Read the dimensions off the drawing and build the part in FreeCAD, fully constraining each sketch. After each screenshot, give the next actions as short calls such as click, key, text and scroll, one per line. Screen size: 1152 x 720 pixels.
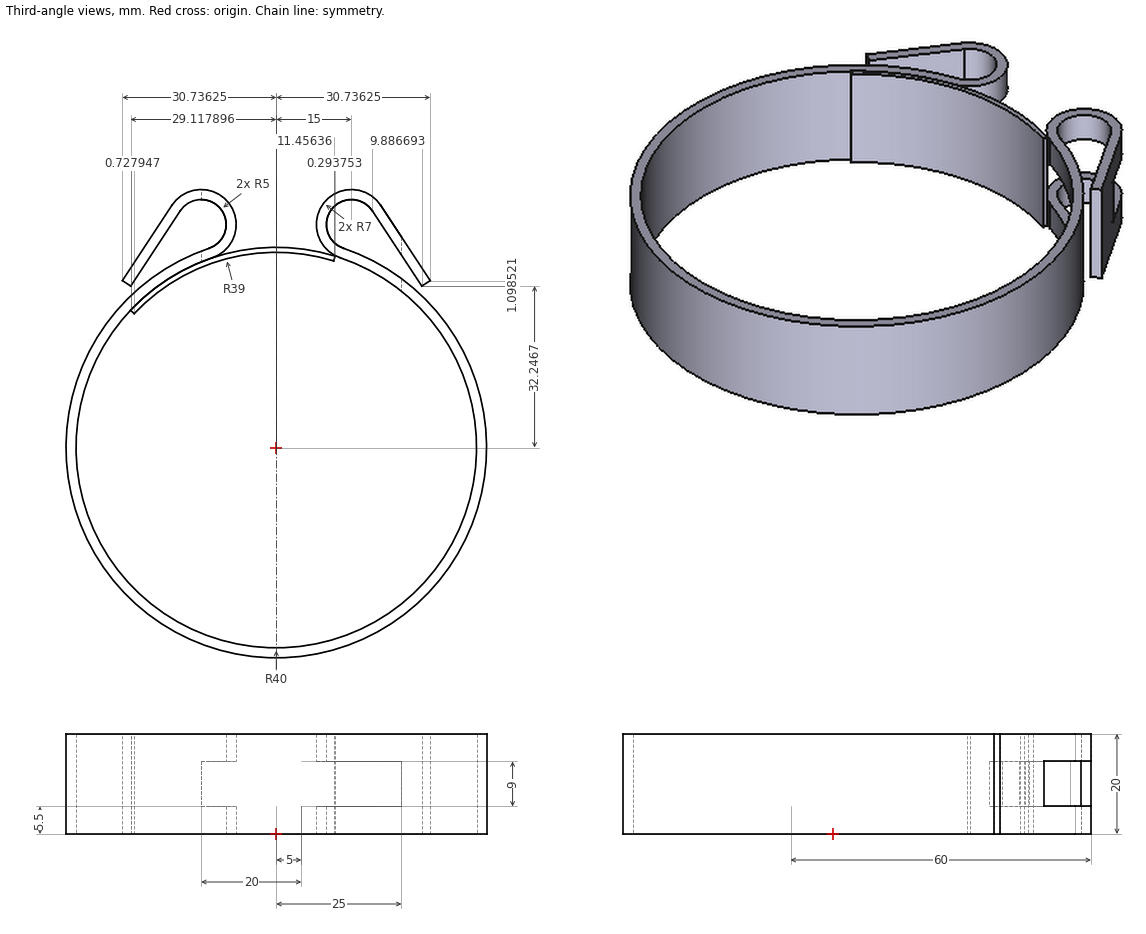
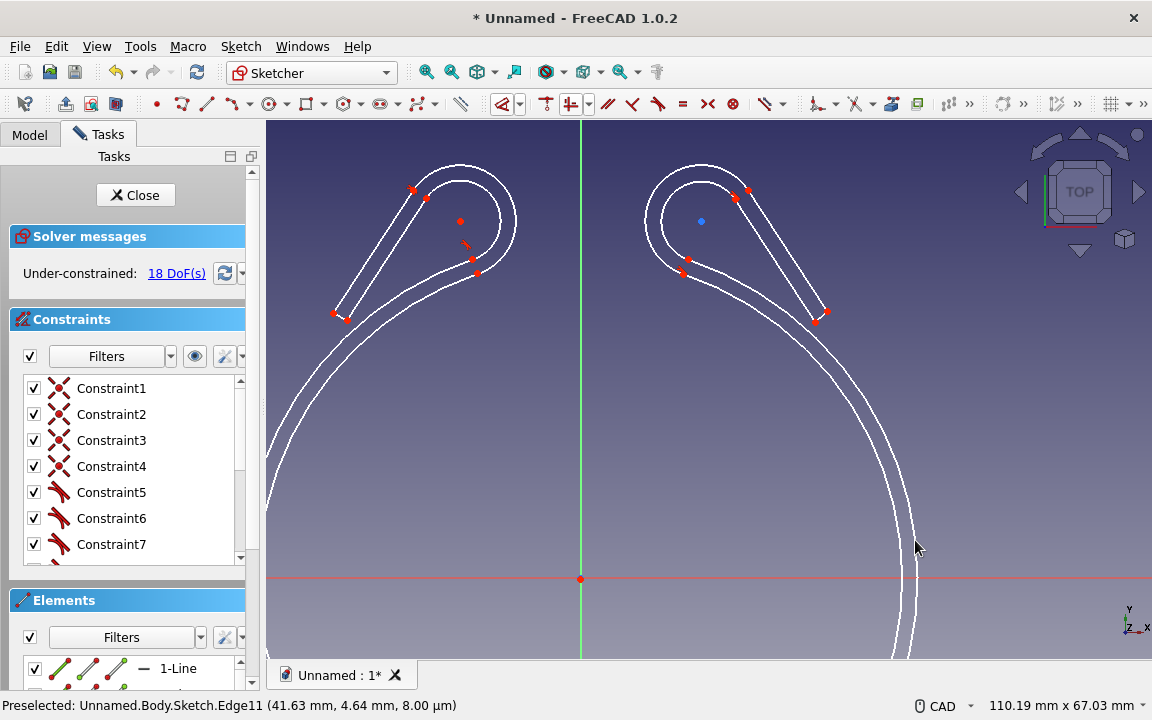
click(693, 166)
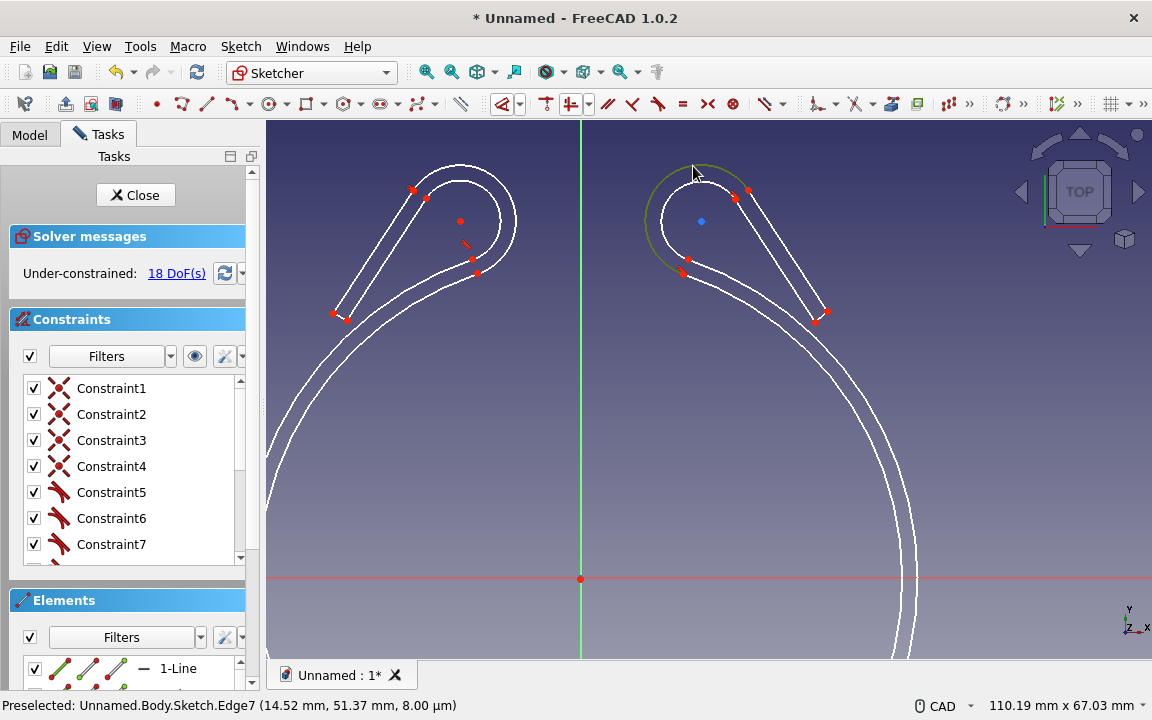
click(696, 182)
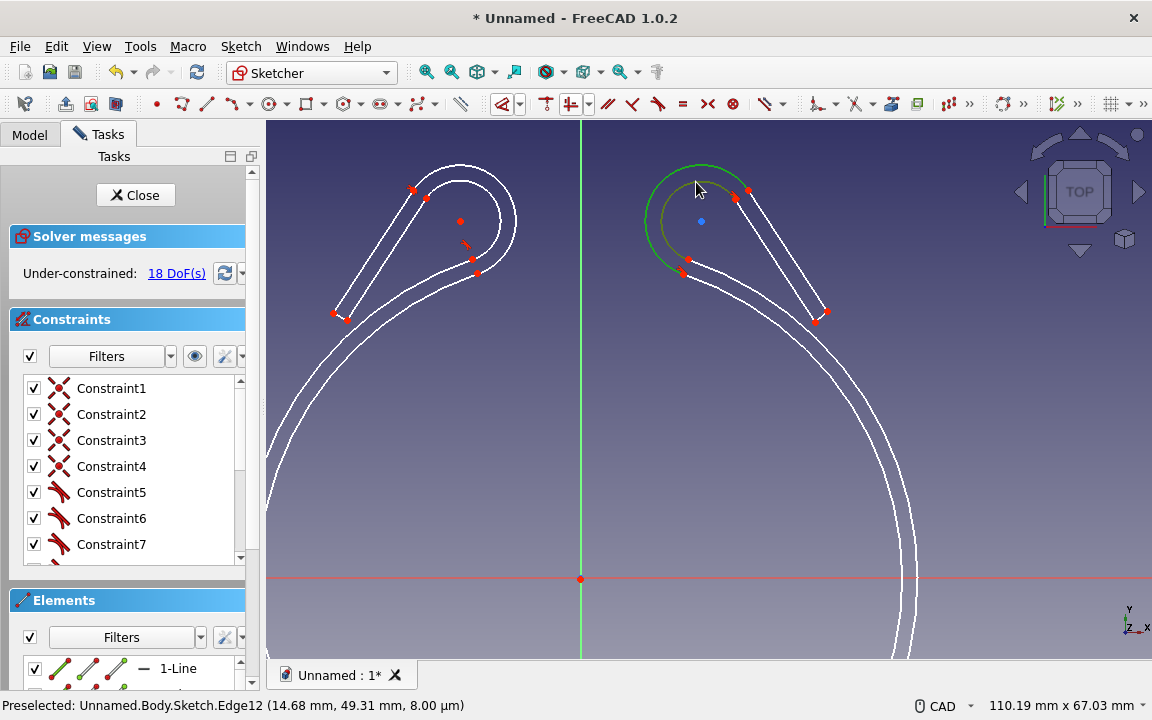
key(c)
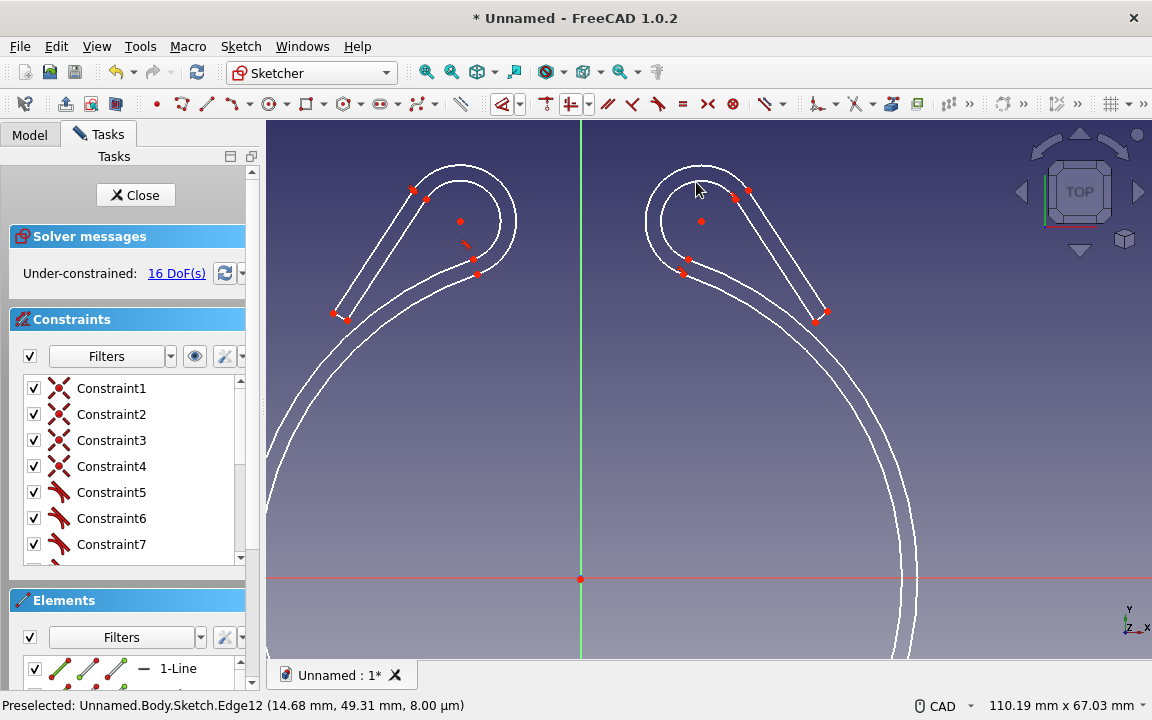
drag(570, 568, 591, 589)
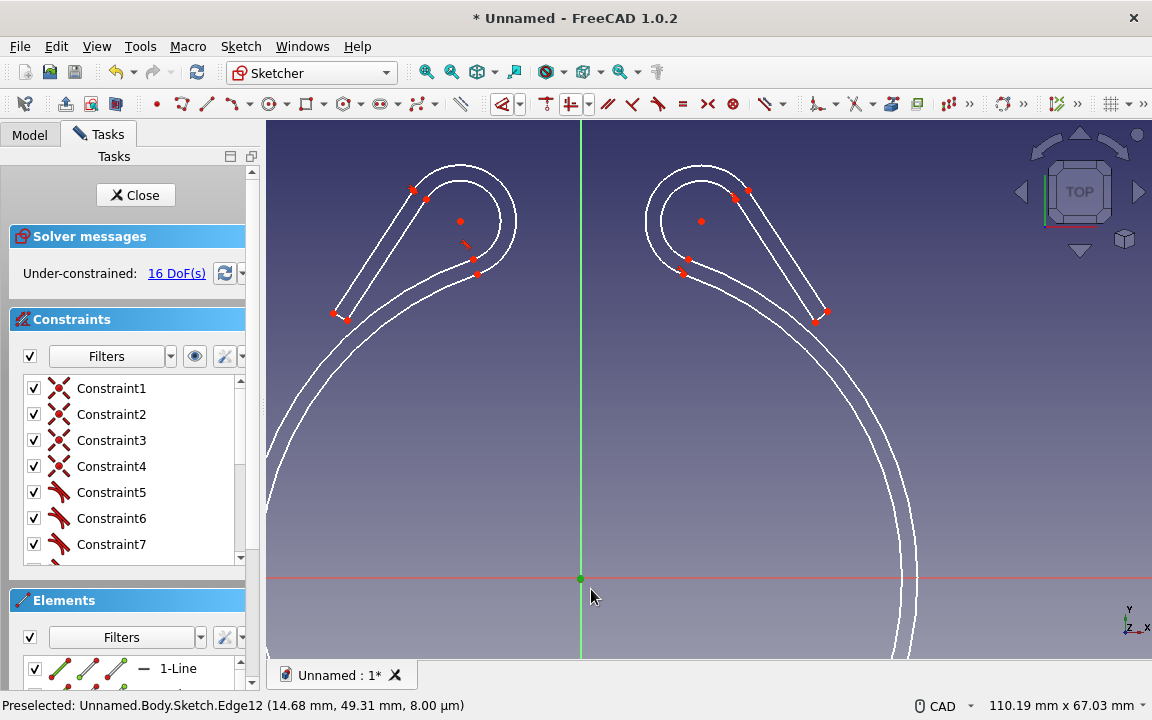
key(c)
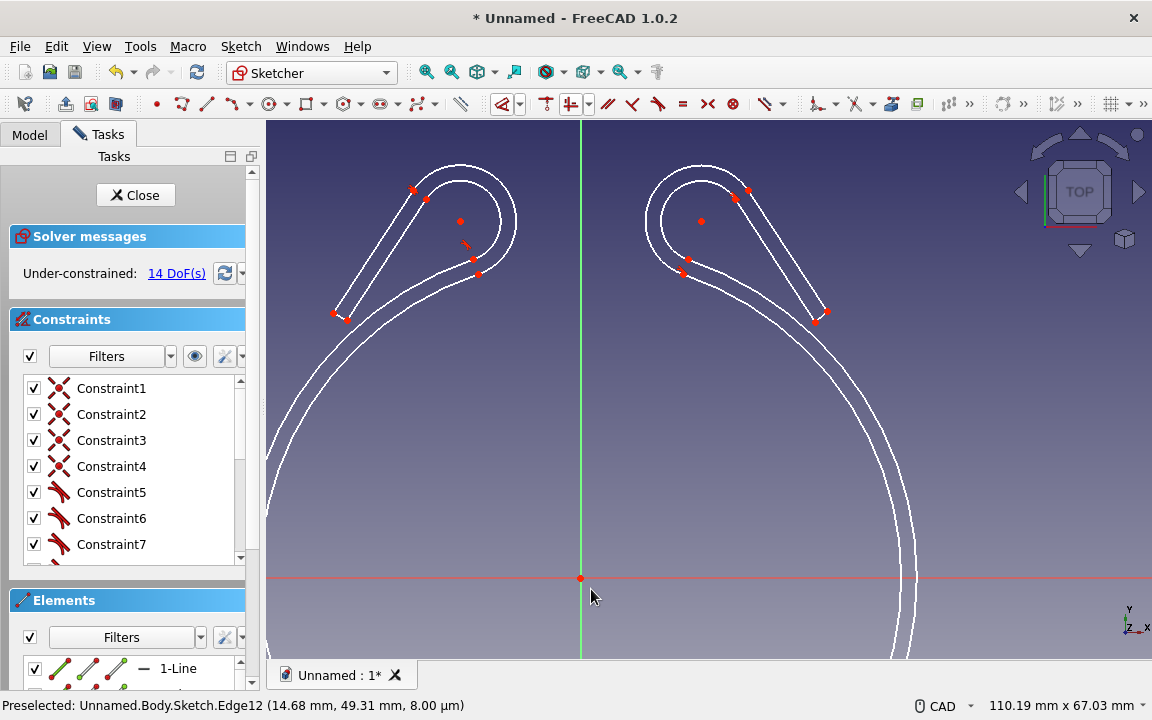
click(693, 166)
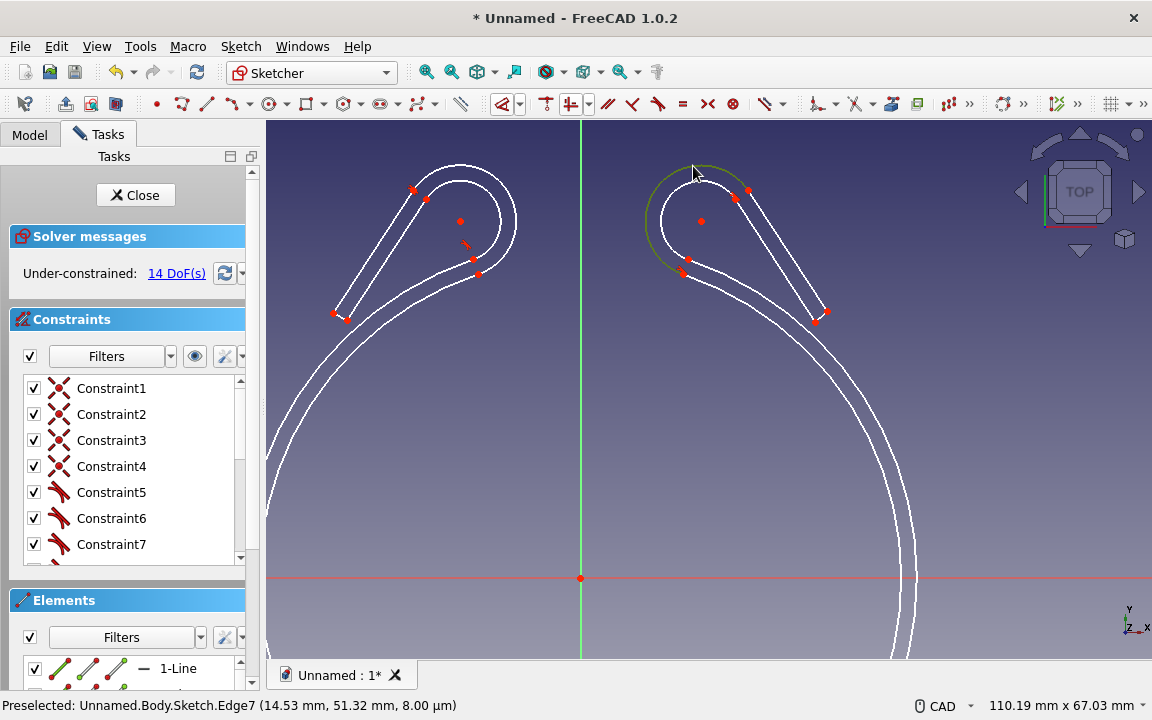
click(516, 227)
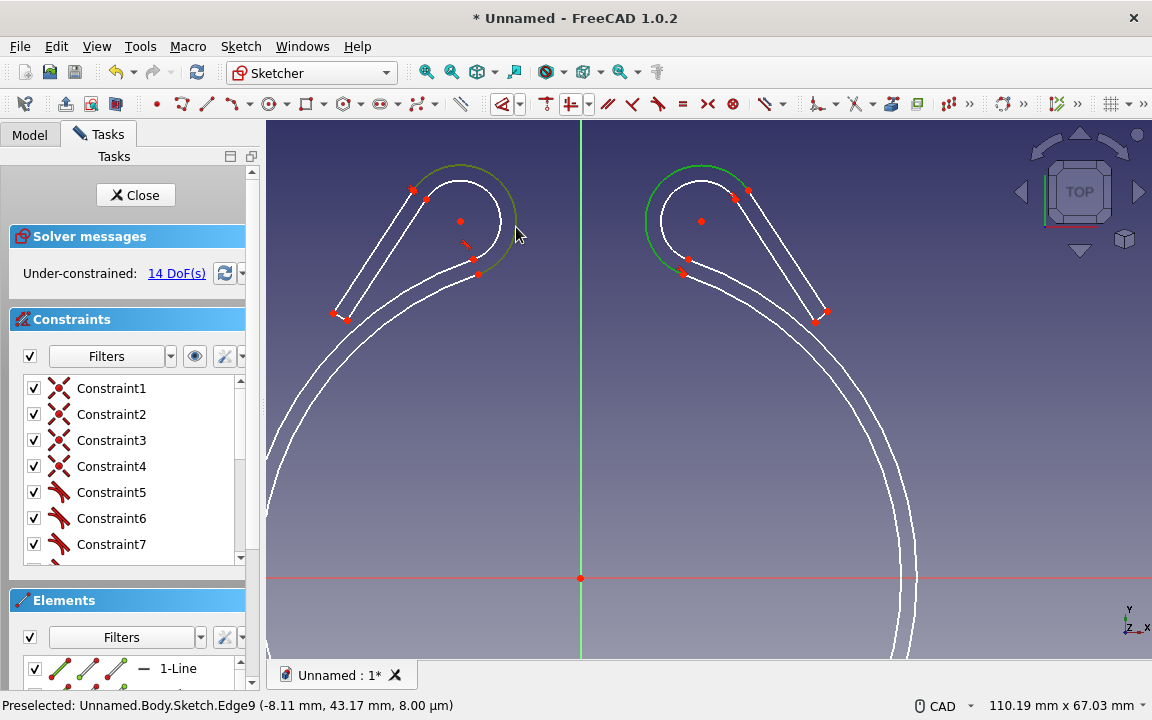
key(e)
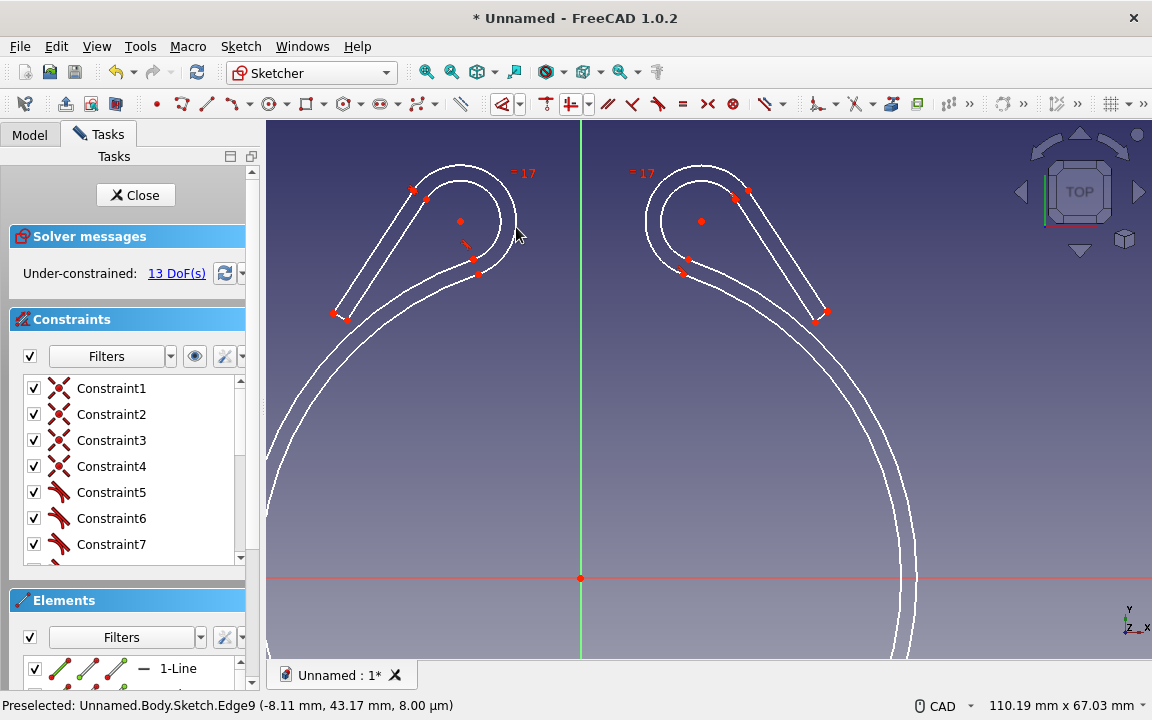
click(748, 191)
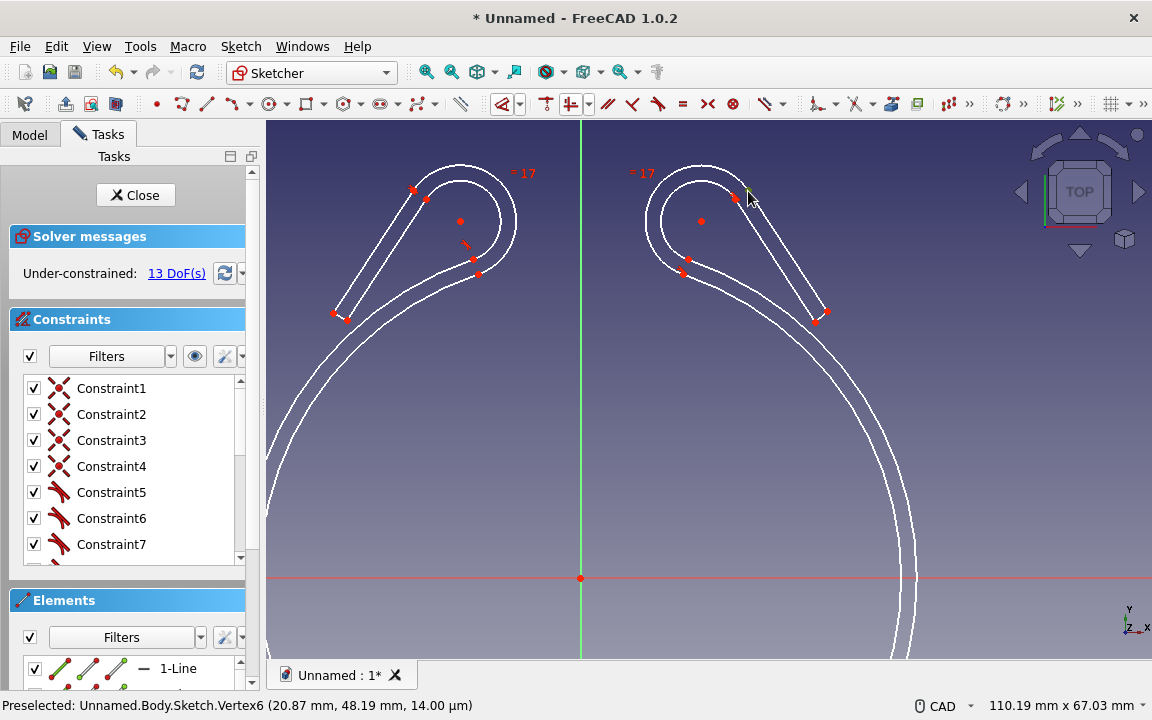
click(413, 191)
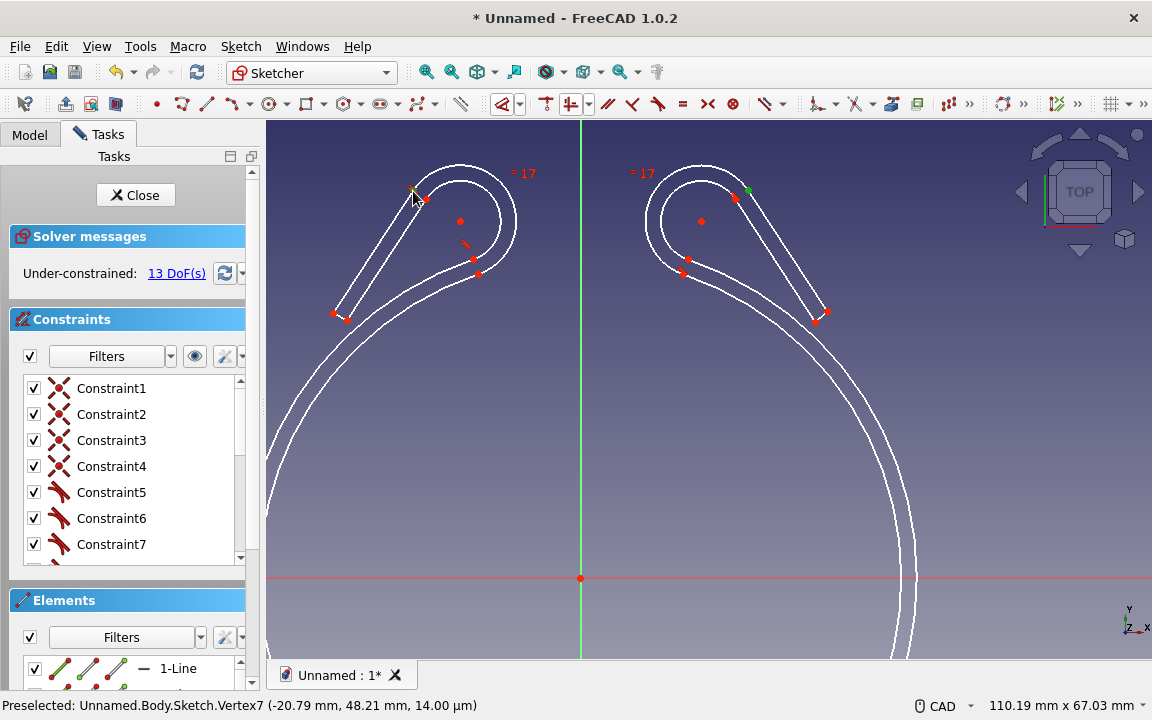
click(581, 528)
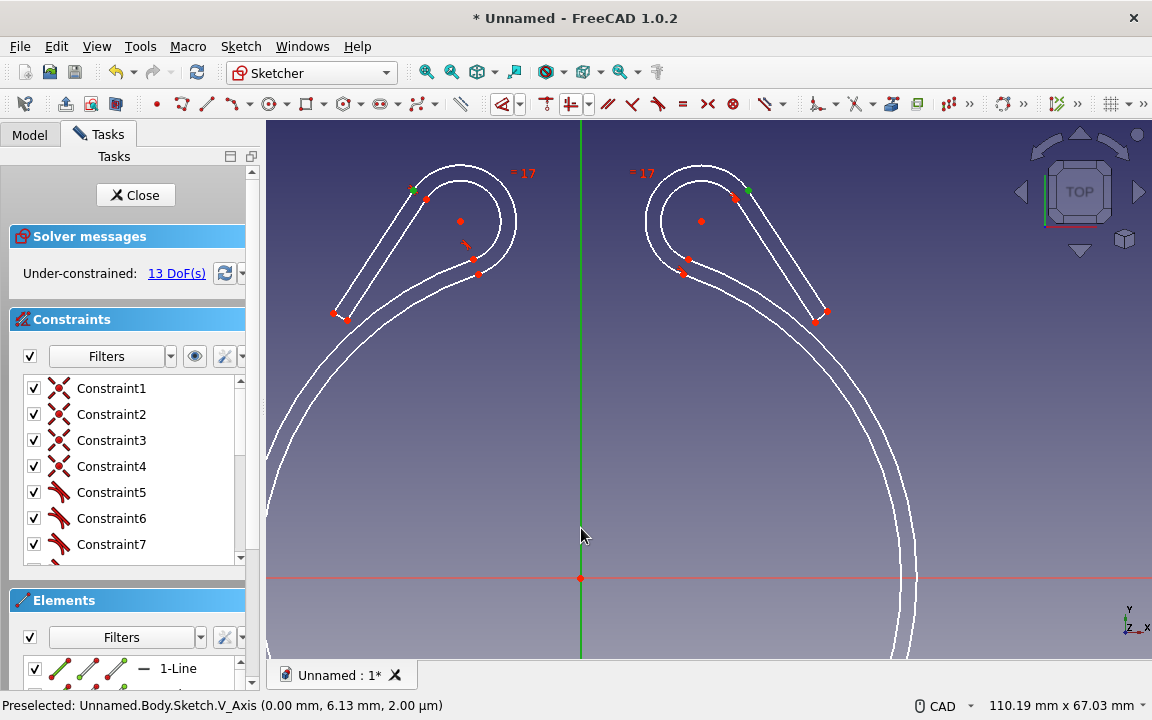
key(s)